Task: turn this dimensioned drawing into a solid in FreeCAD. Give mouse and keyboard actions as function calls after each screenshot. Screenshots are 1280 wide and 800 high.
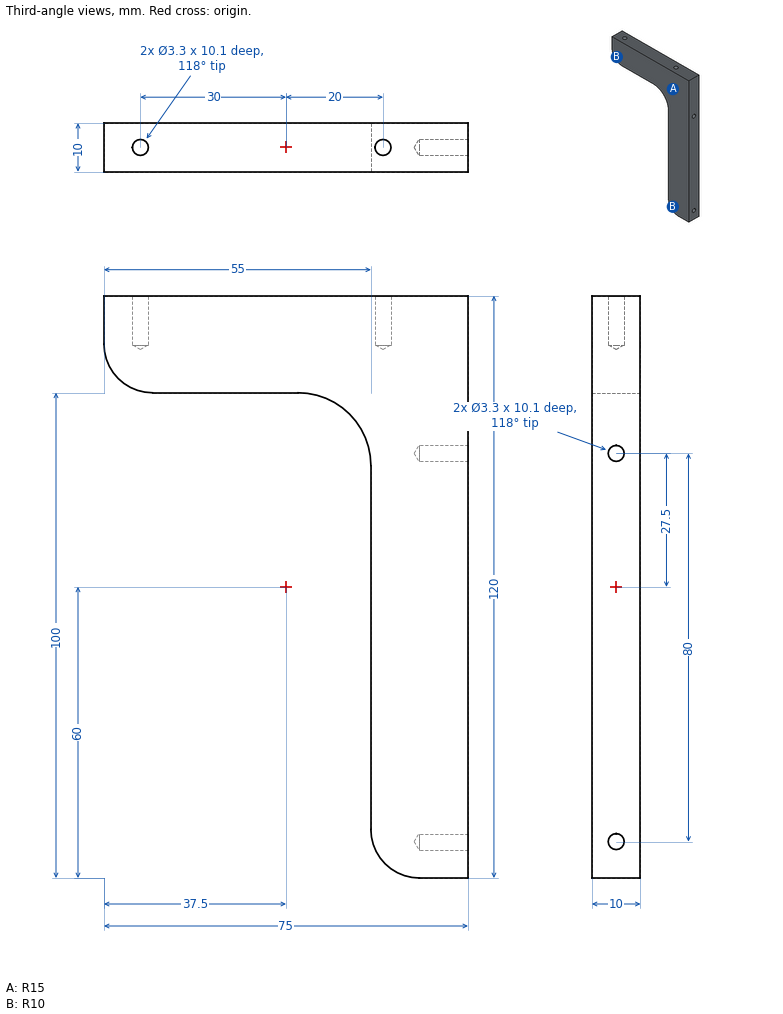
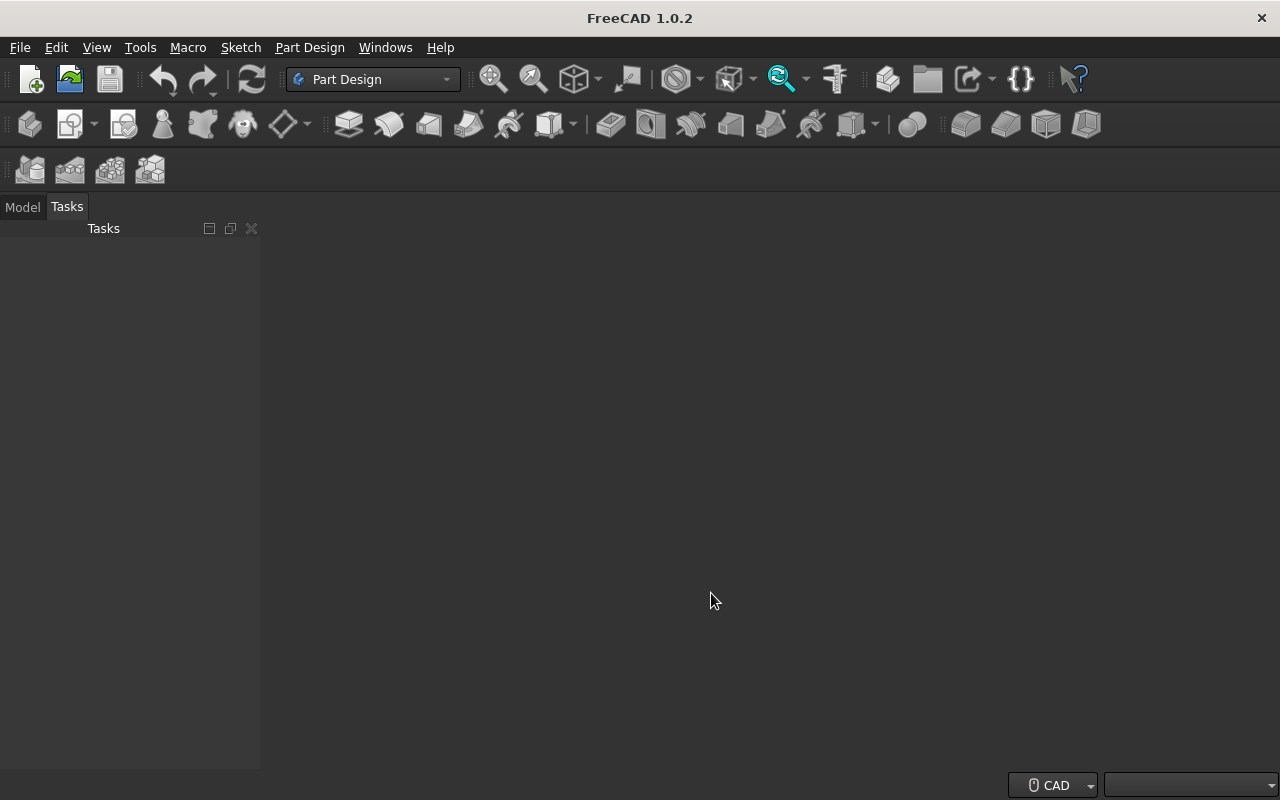
click(30, 80)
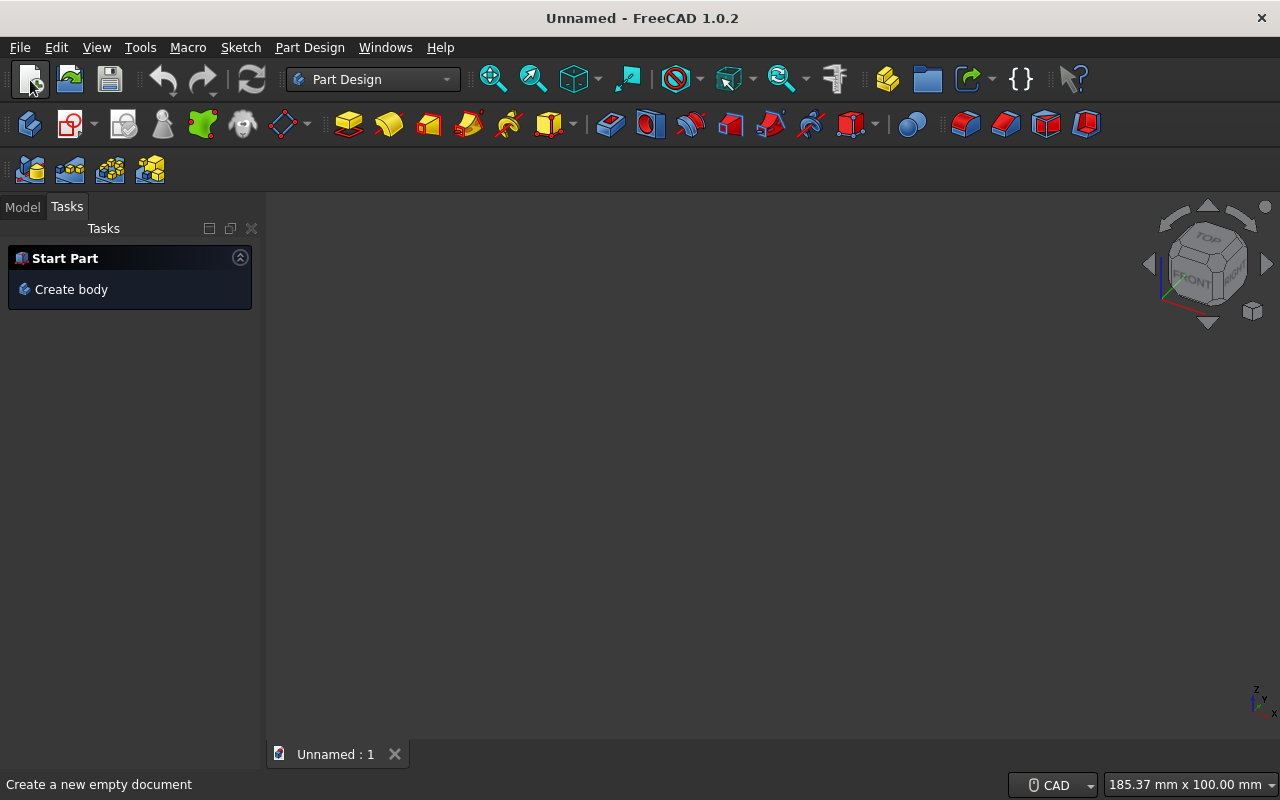
click(70, 124)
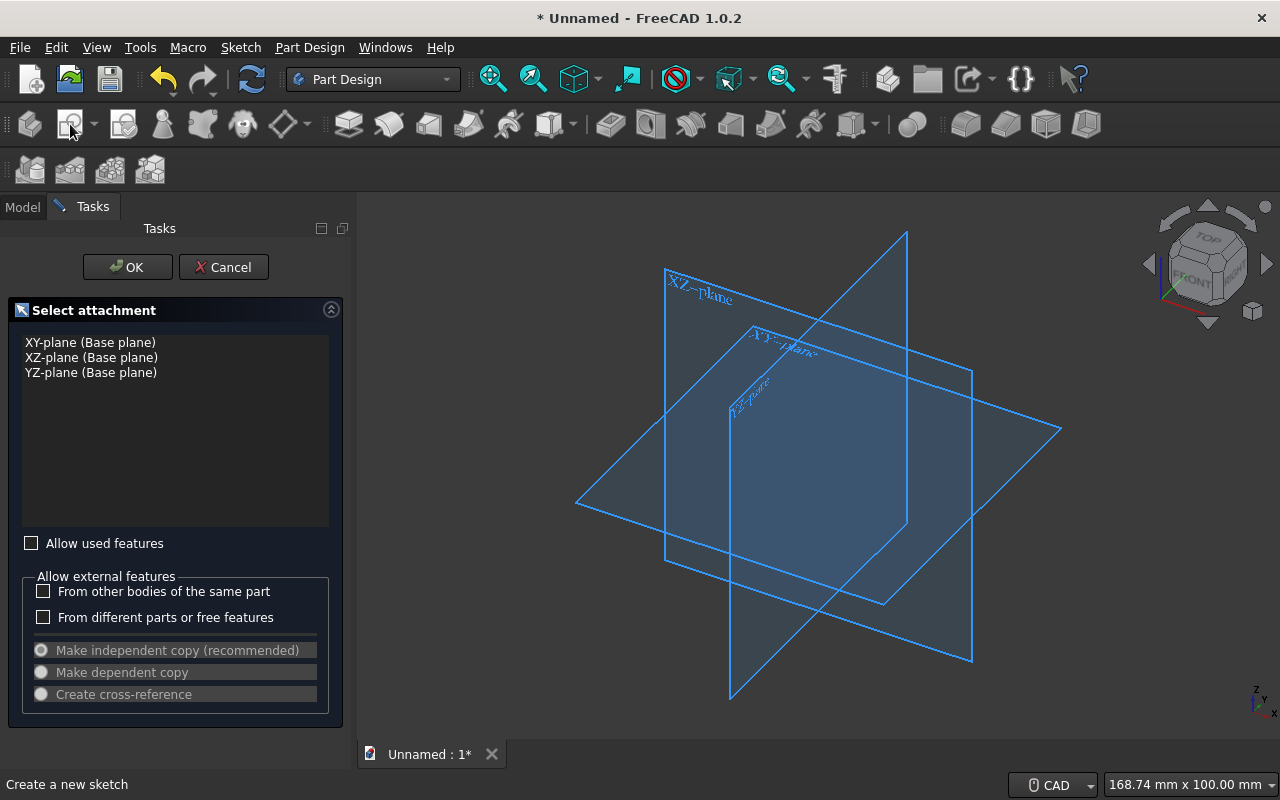
click(82, 358)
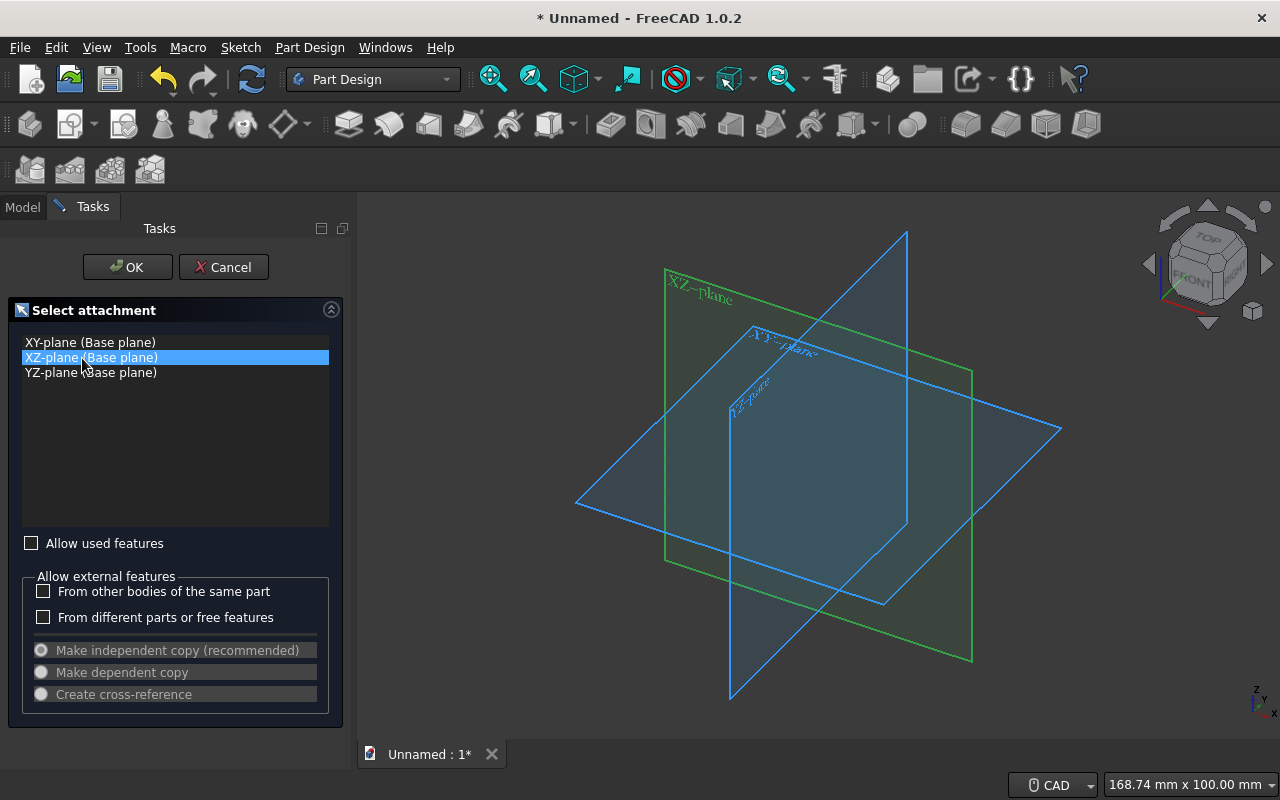
click(128, 267)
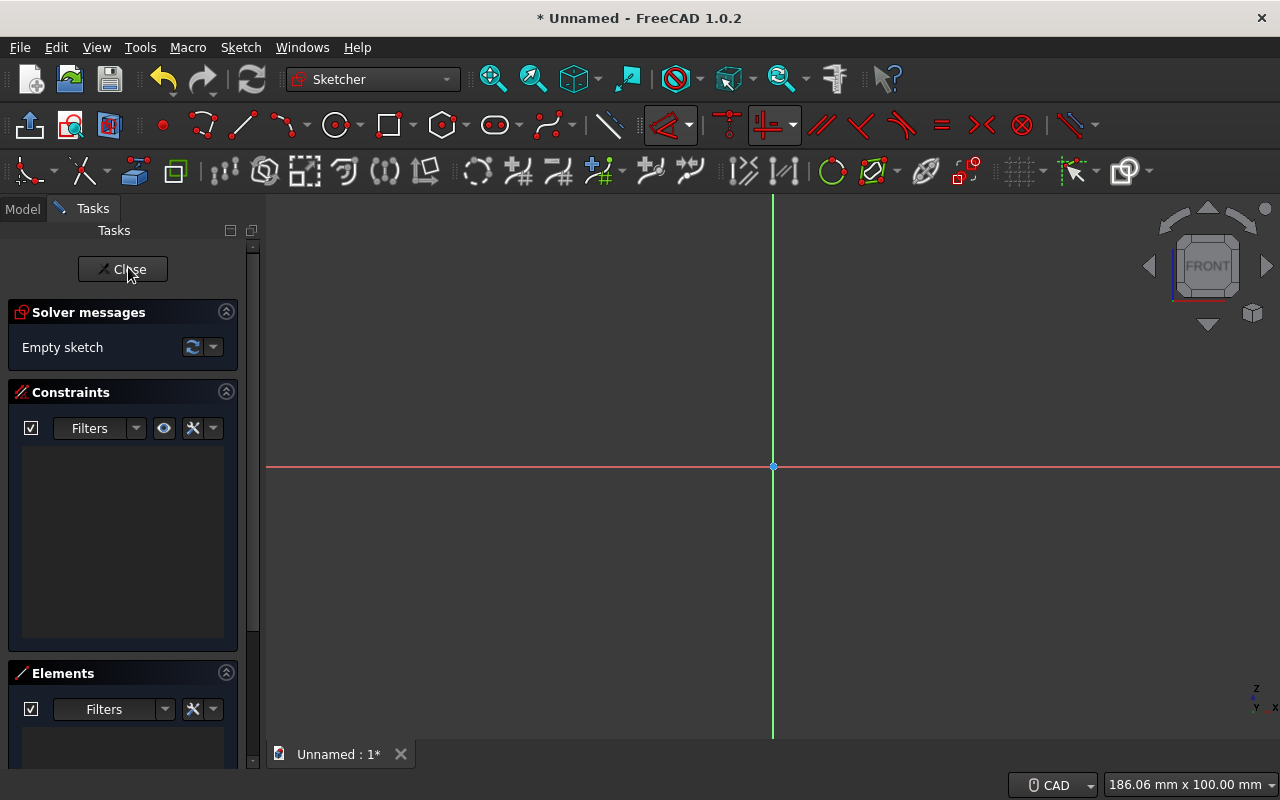
scroll(621, 466, down, 3)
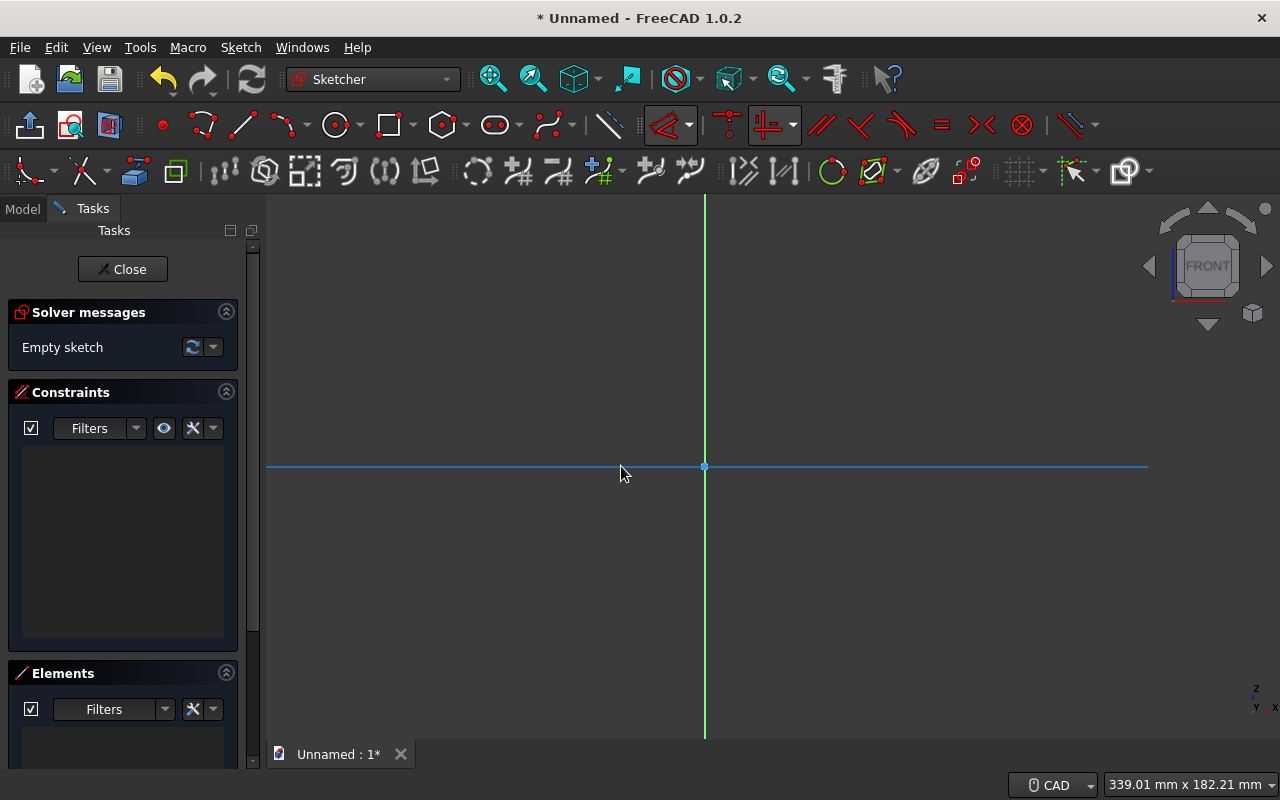
key(g)
key(v)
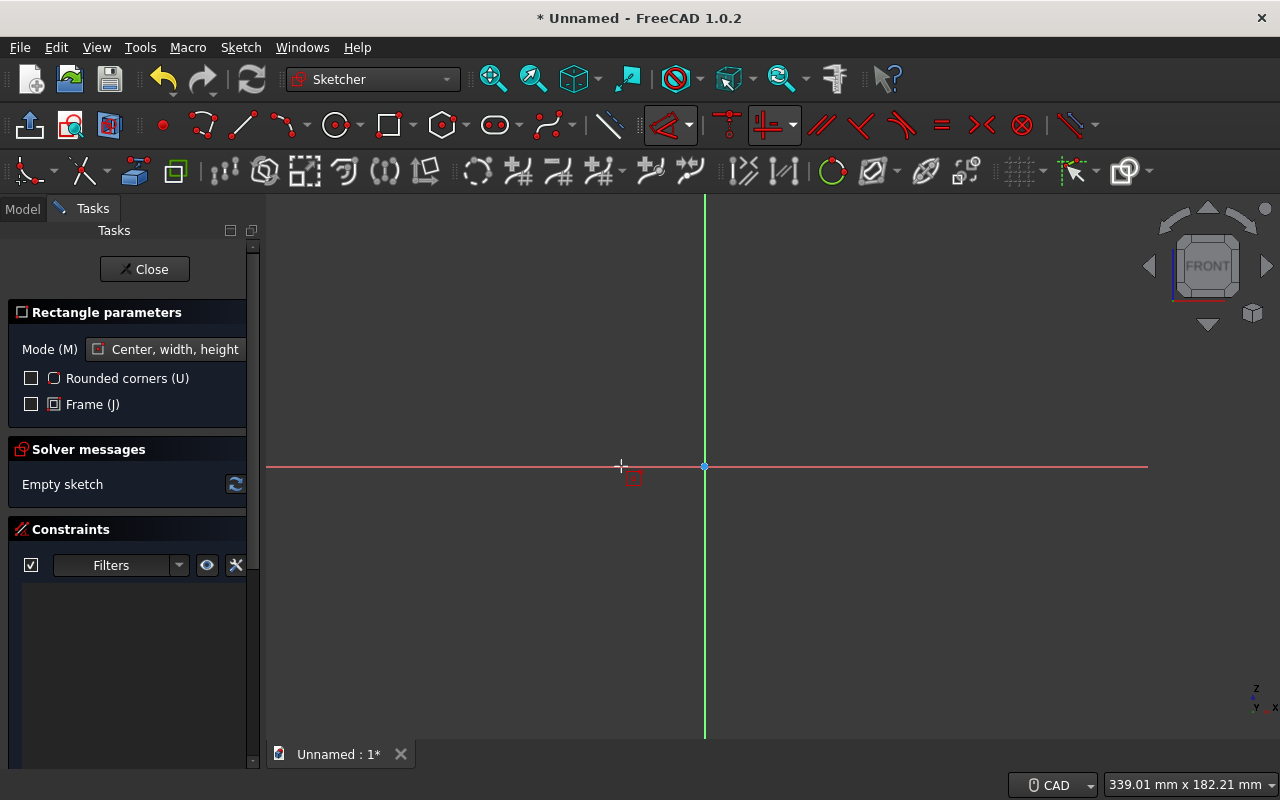
click(705, 466)
click(817, 287)
key(Escape)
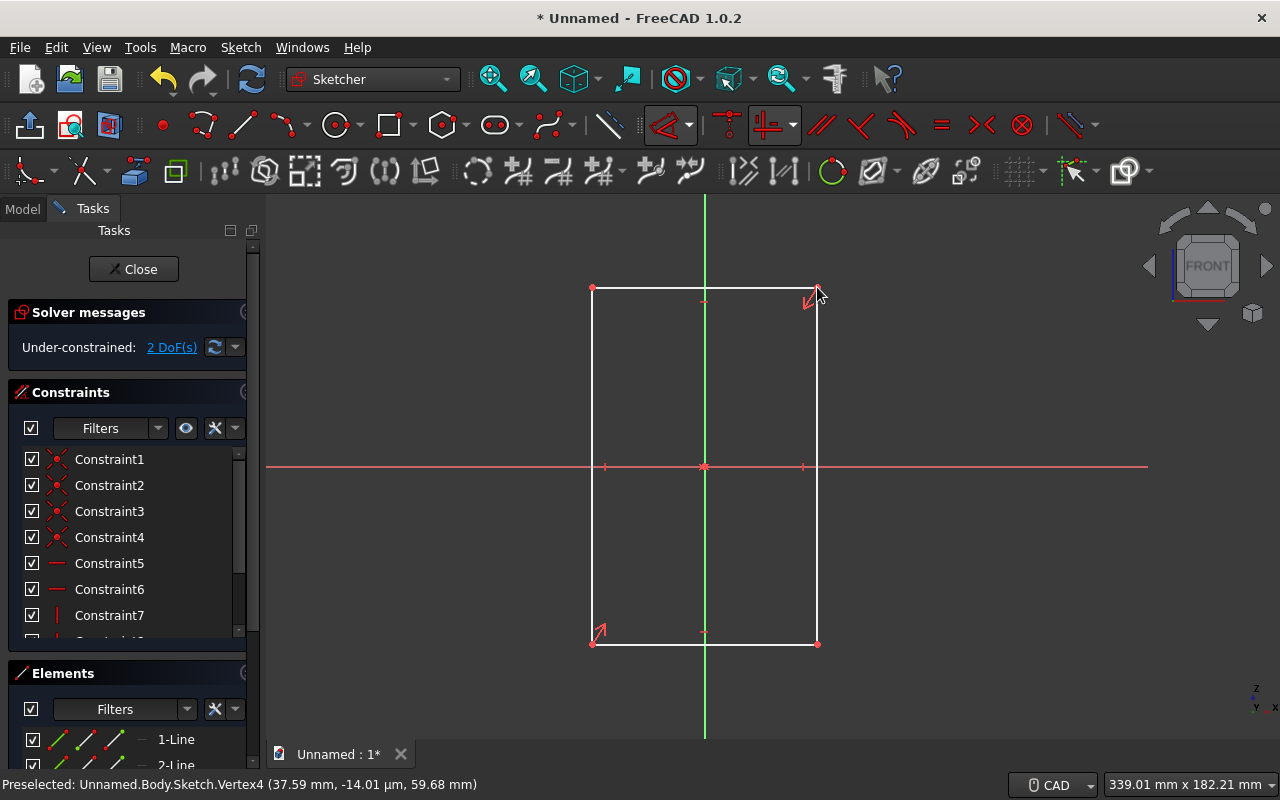
key(d)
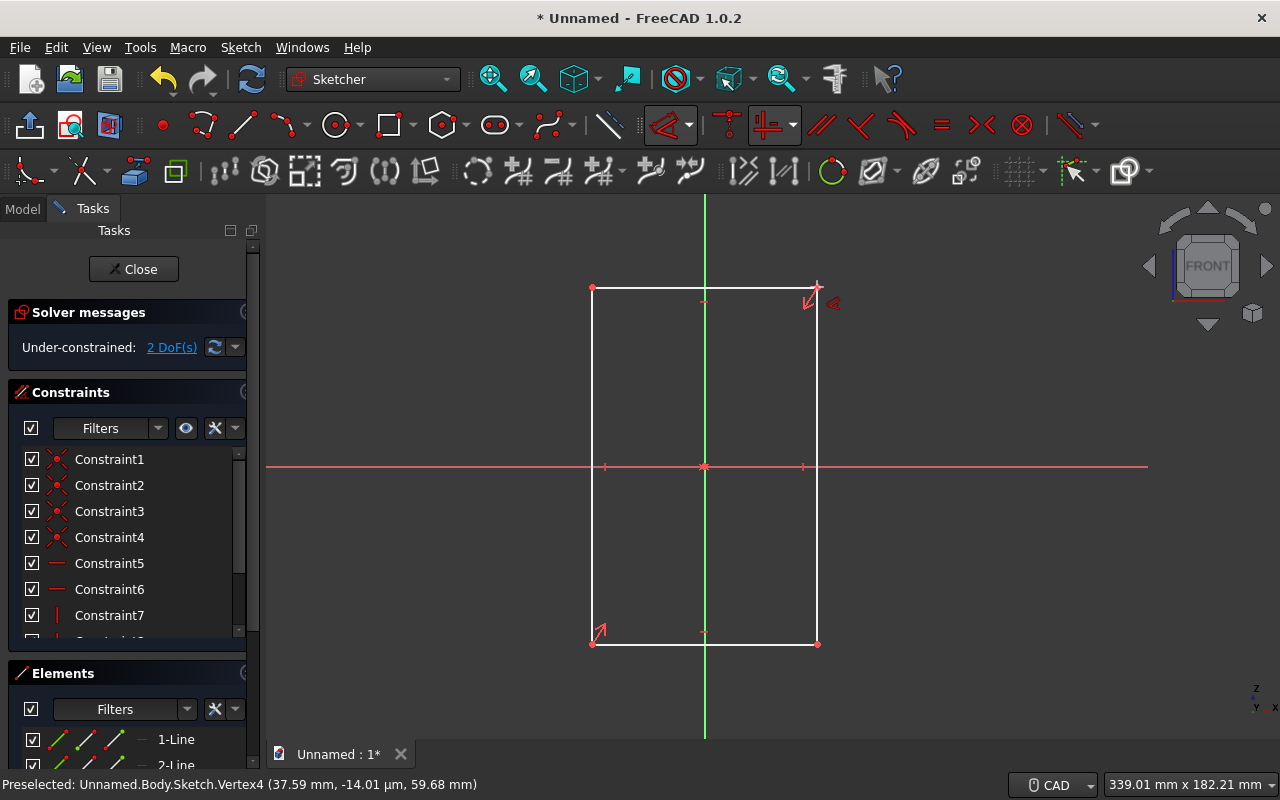
click(660, 645)
click(653, 679)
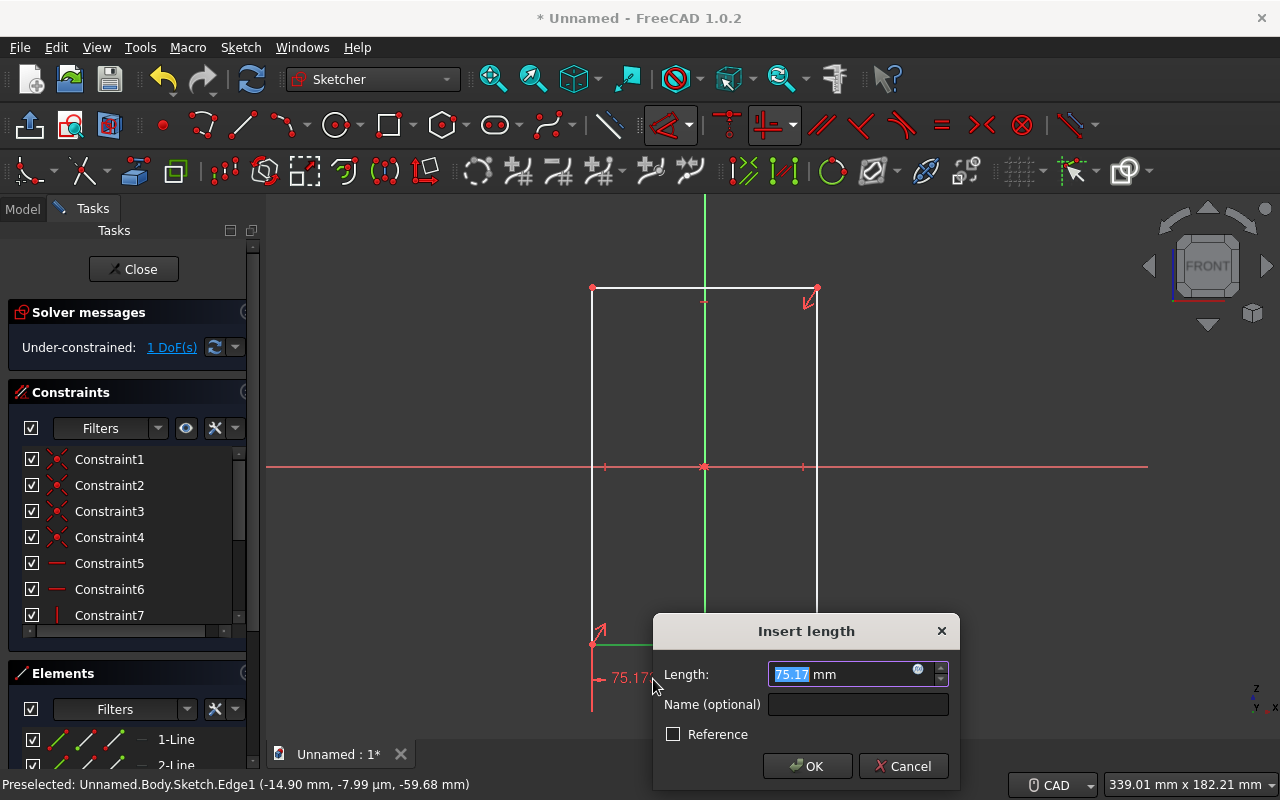
text(75)
key(Return)